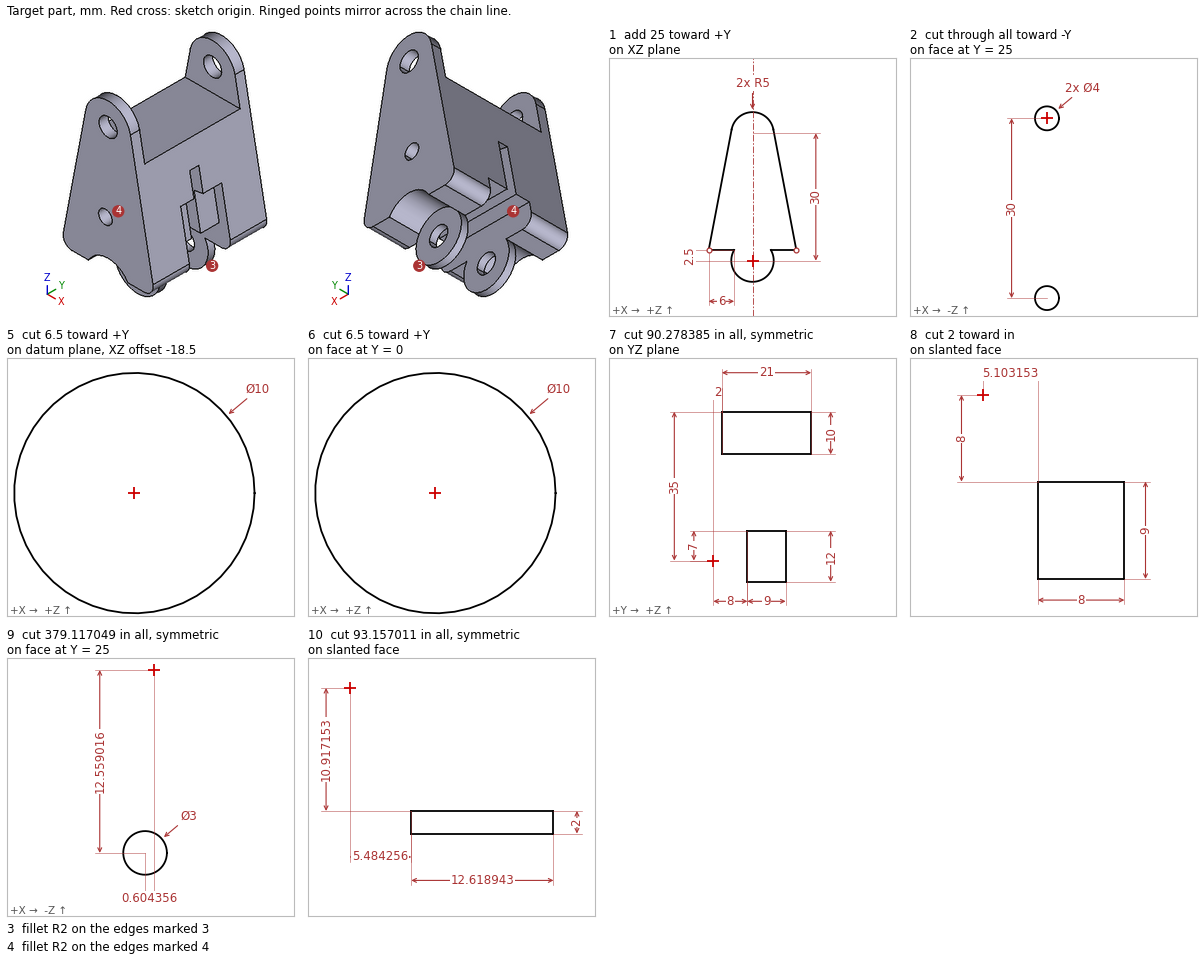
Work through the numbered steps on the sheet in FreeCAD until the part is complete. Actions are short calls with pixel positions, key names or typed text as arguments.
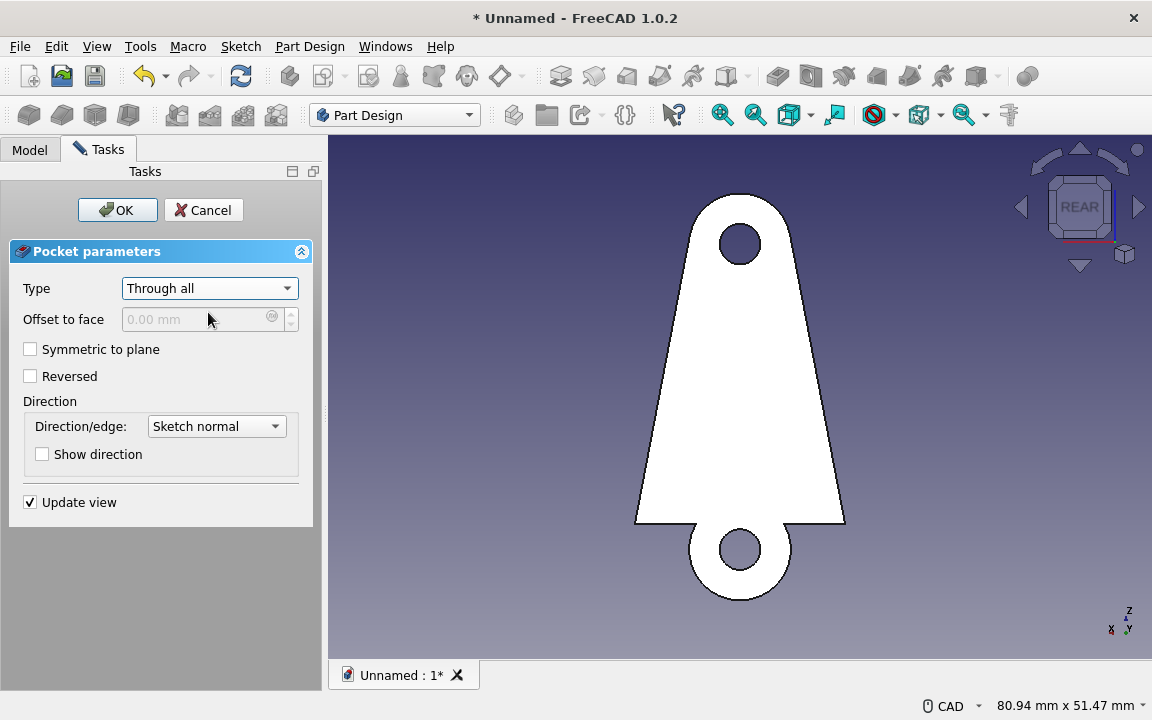
click(118, 210)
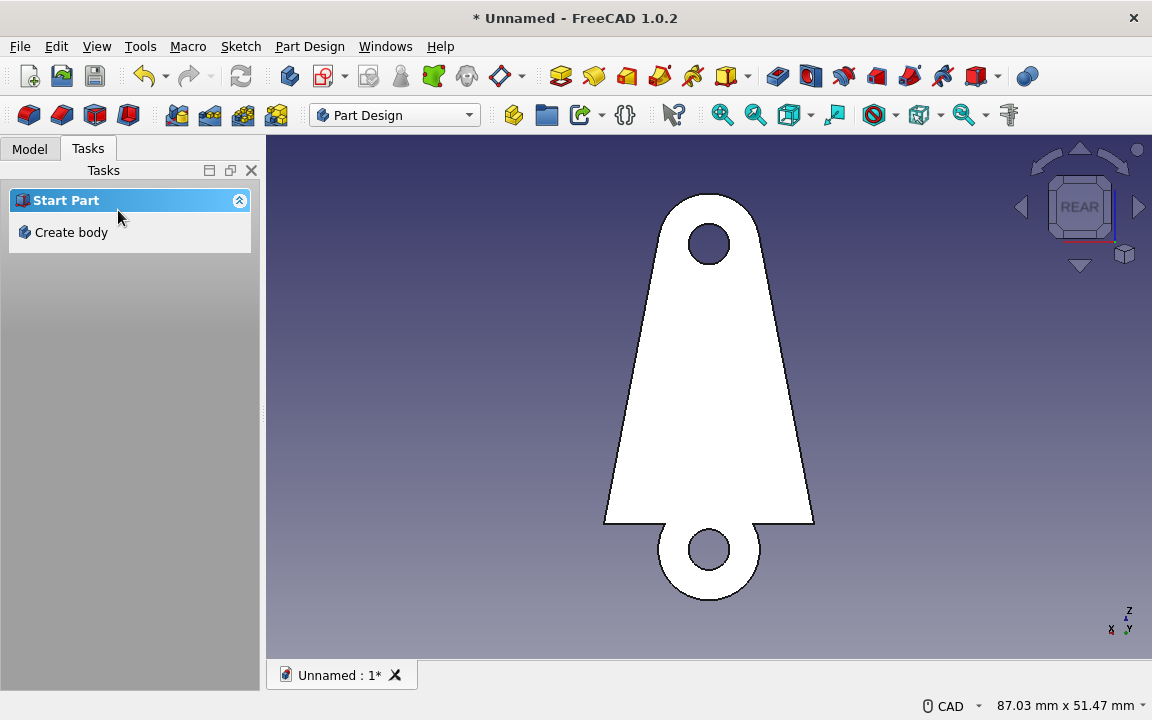
key(0)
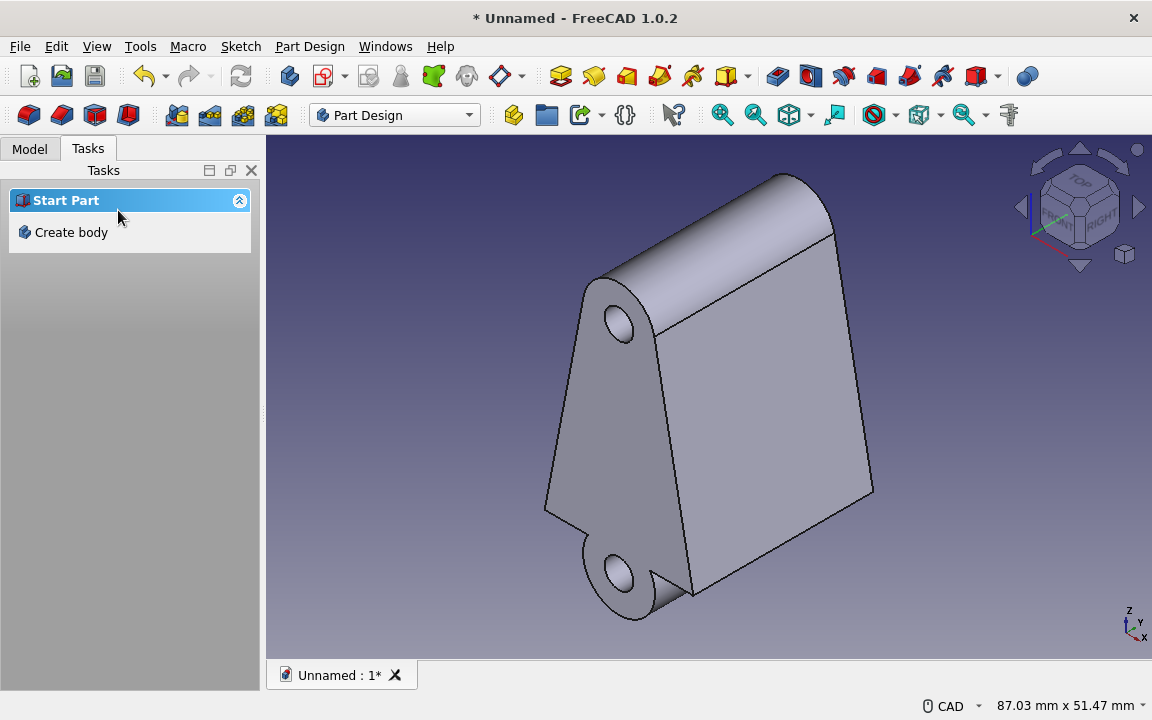
key(2)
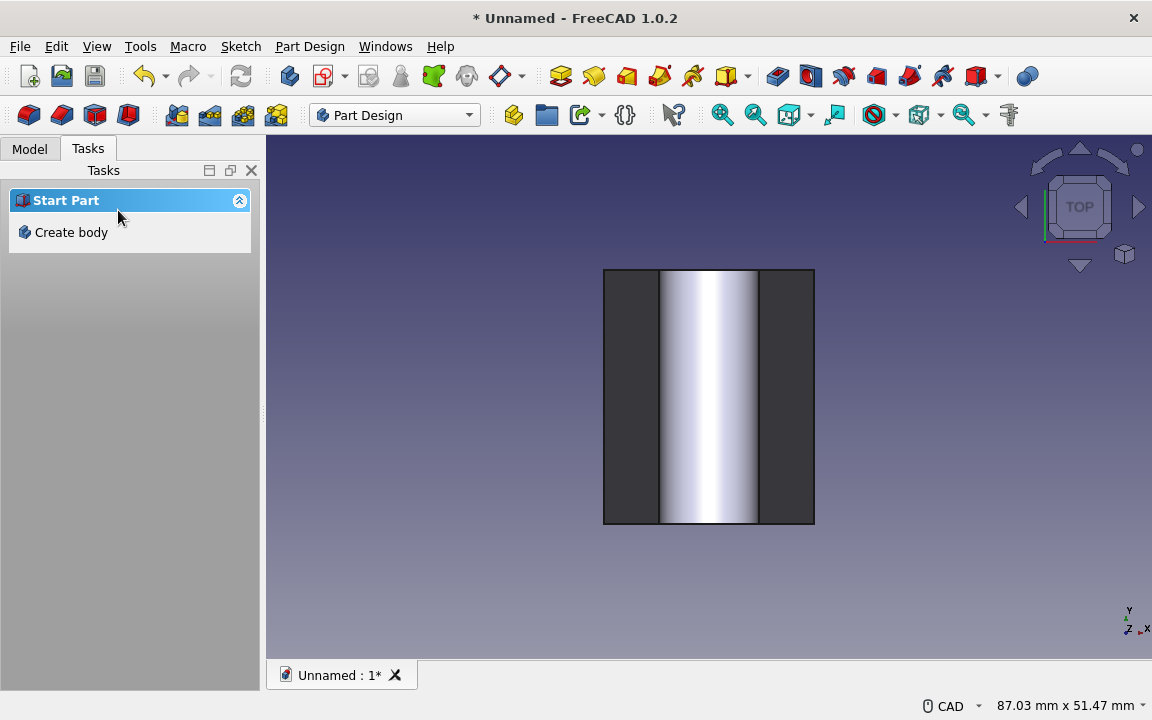
key(1)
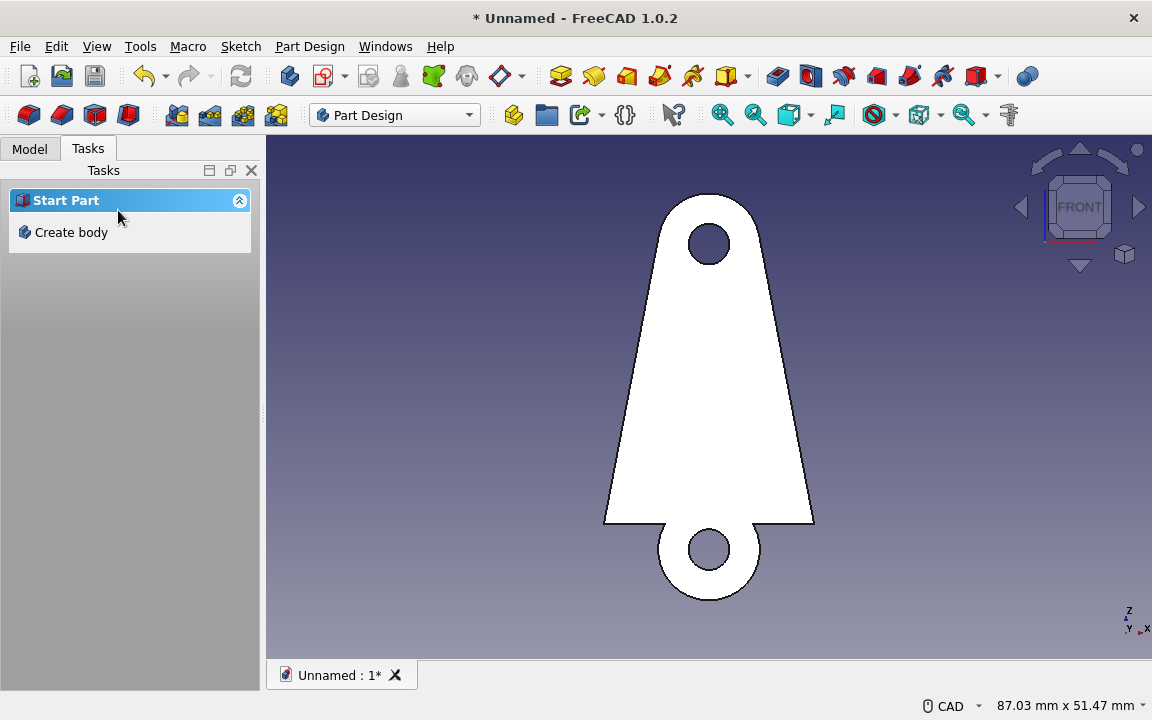
key(3)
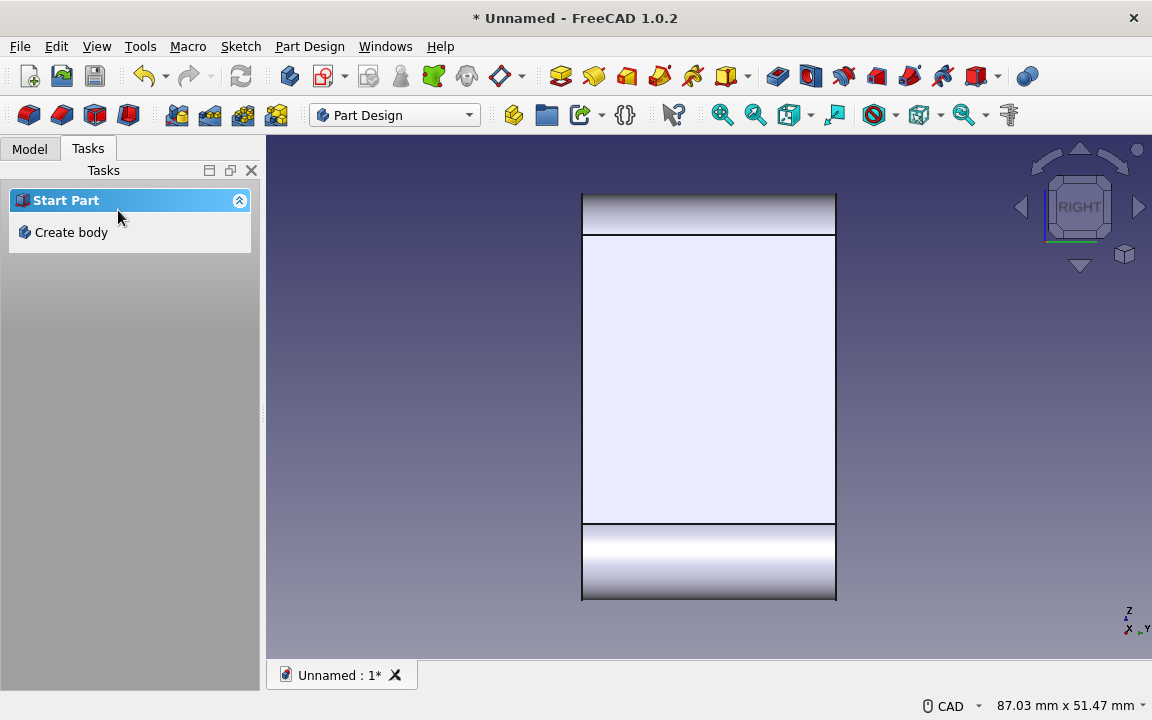
click(709, 523)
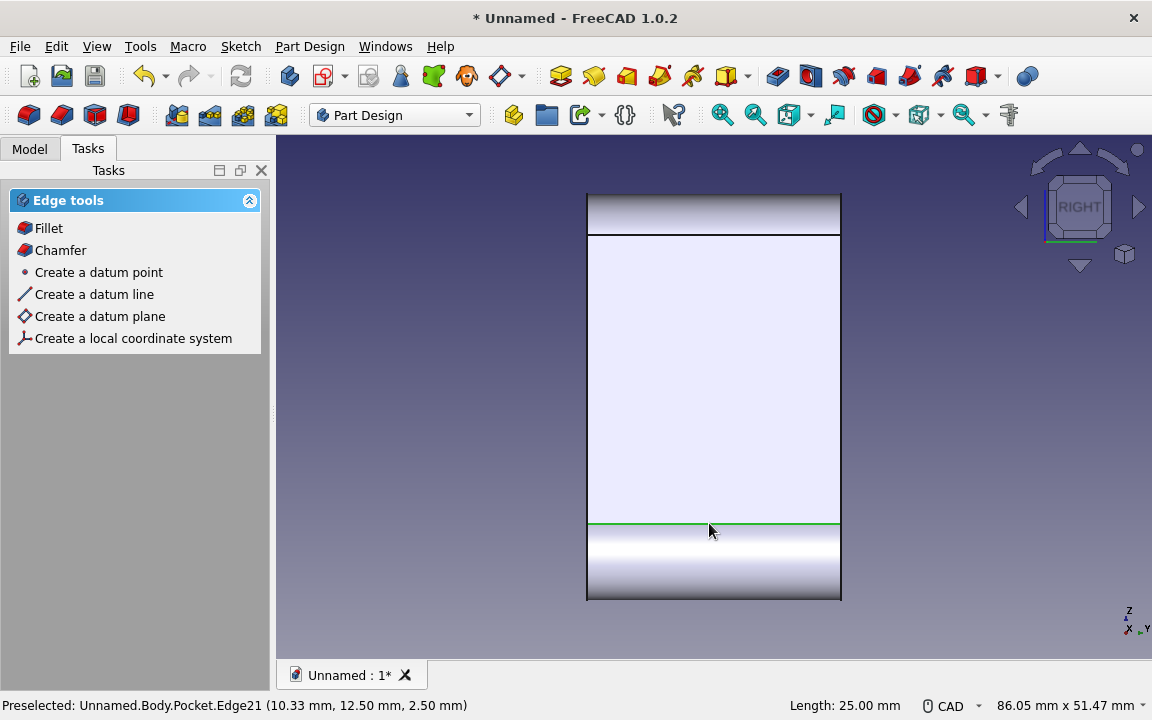
click(29, 116)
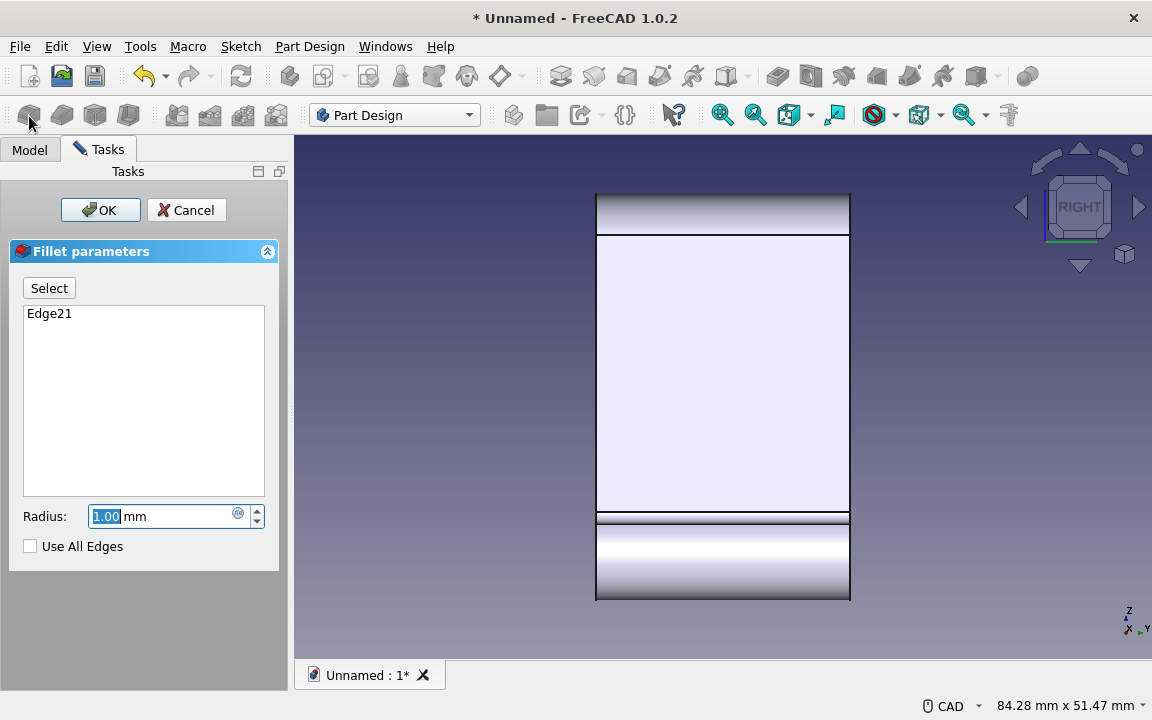
text(2)
key(Tab)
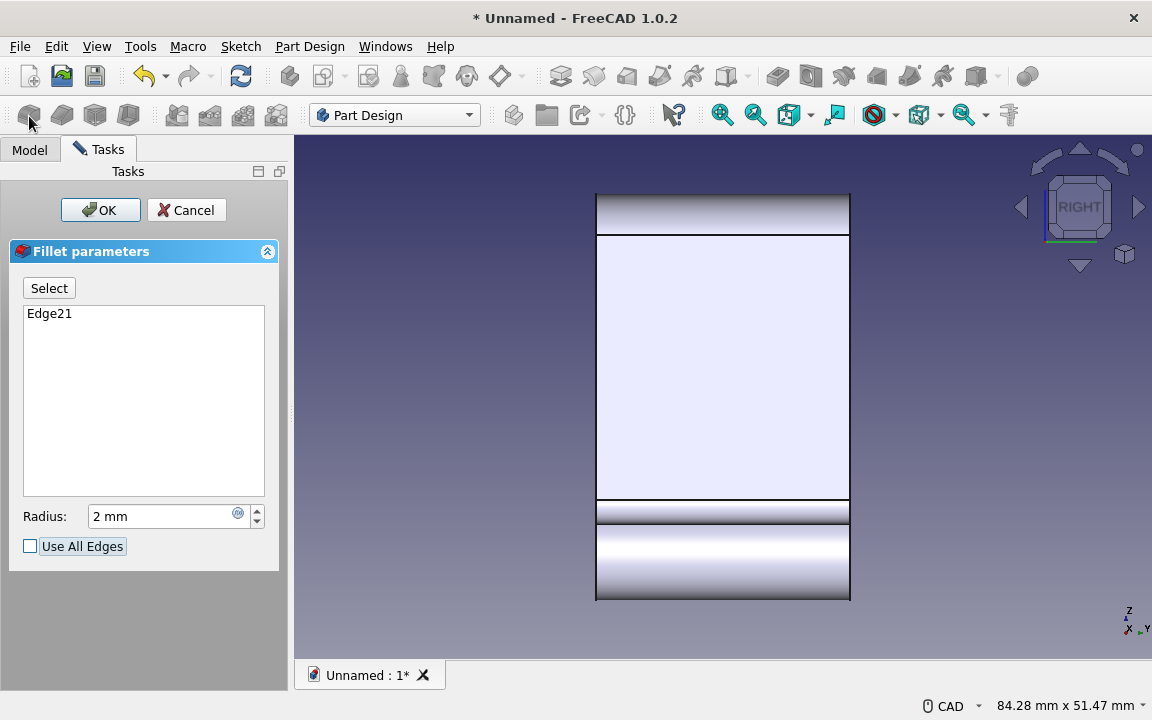
click(101, 210)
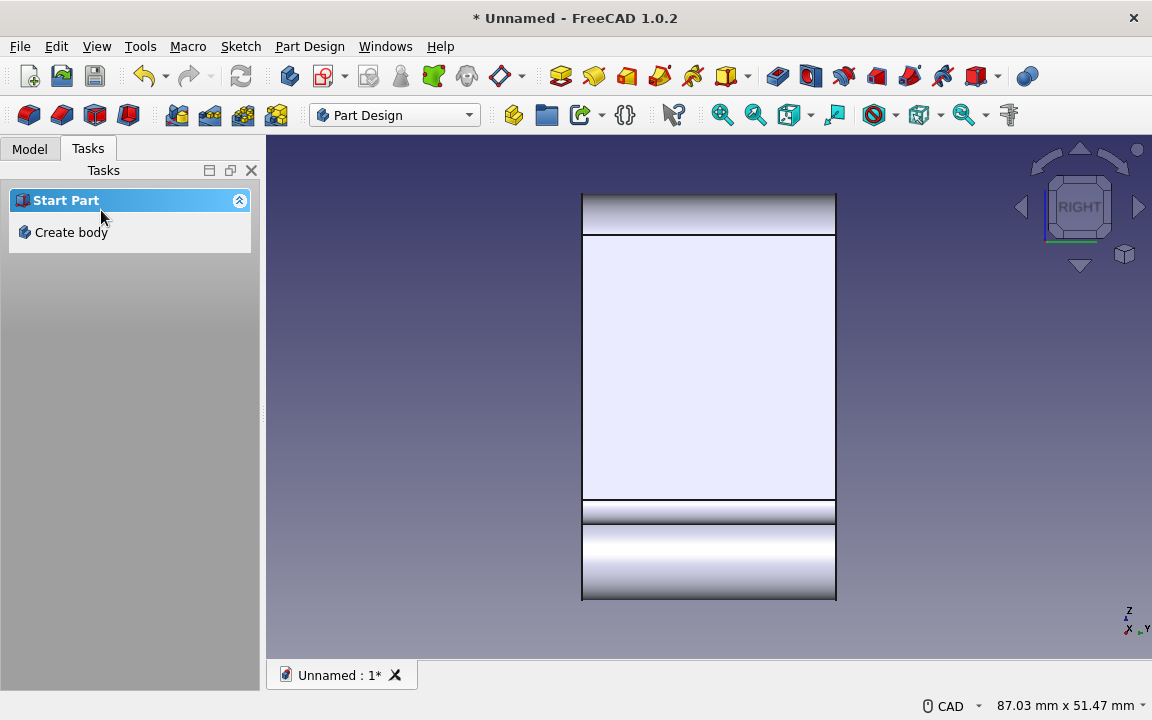
key(0)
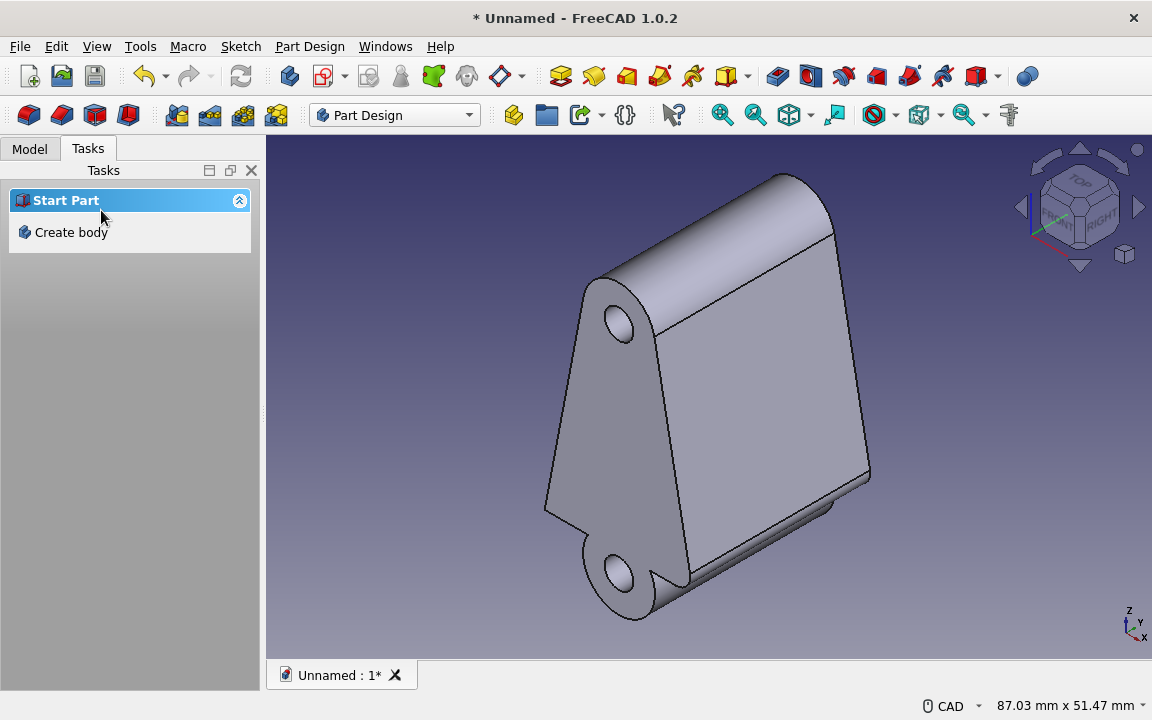
key(2)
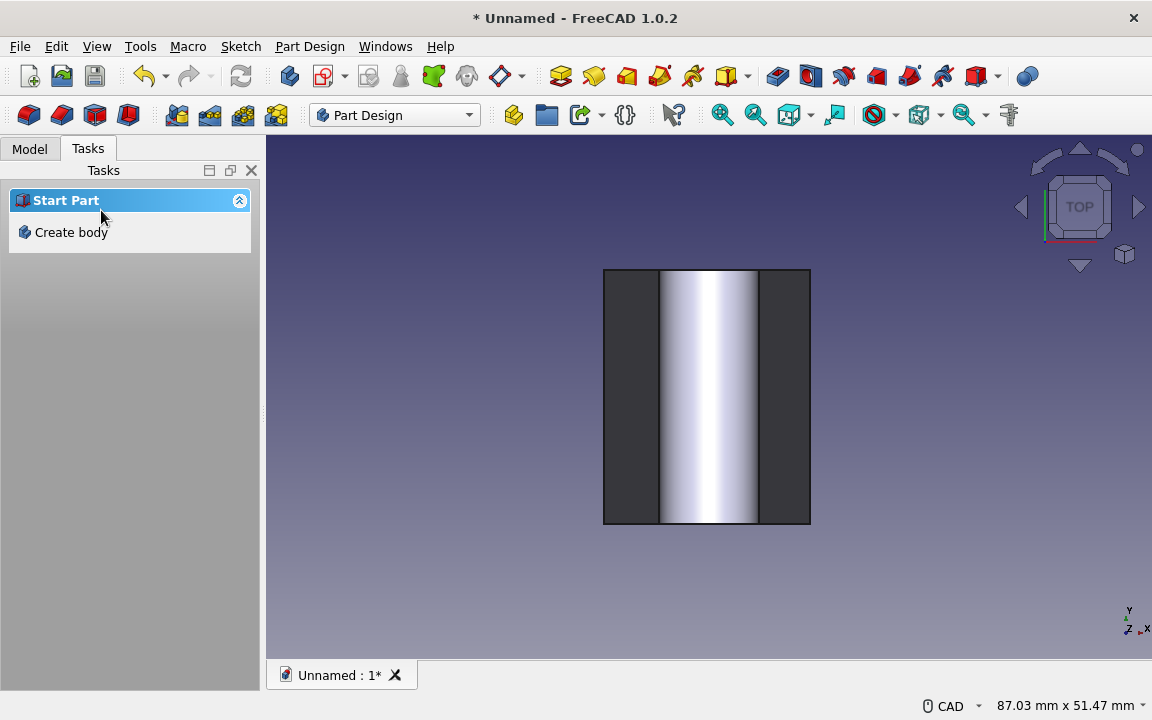
key(1)